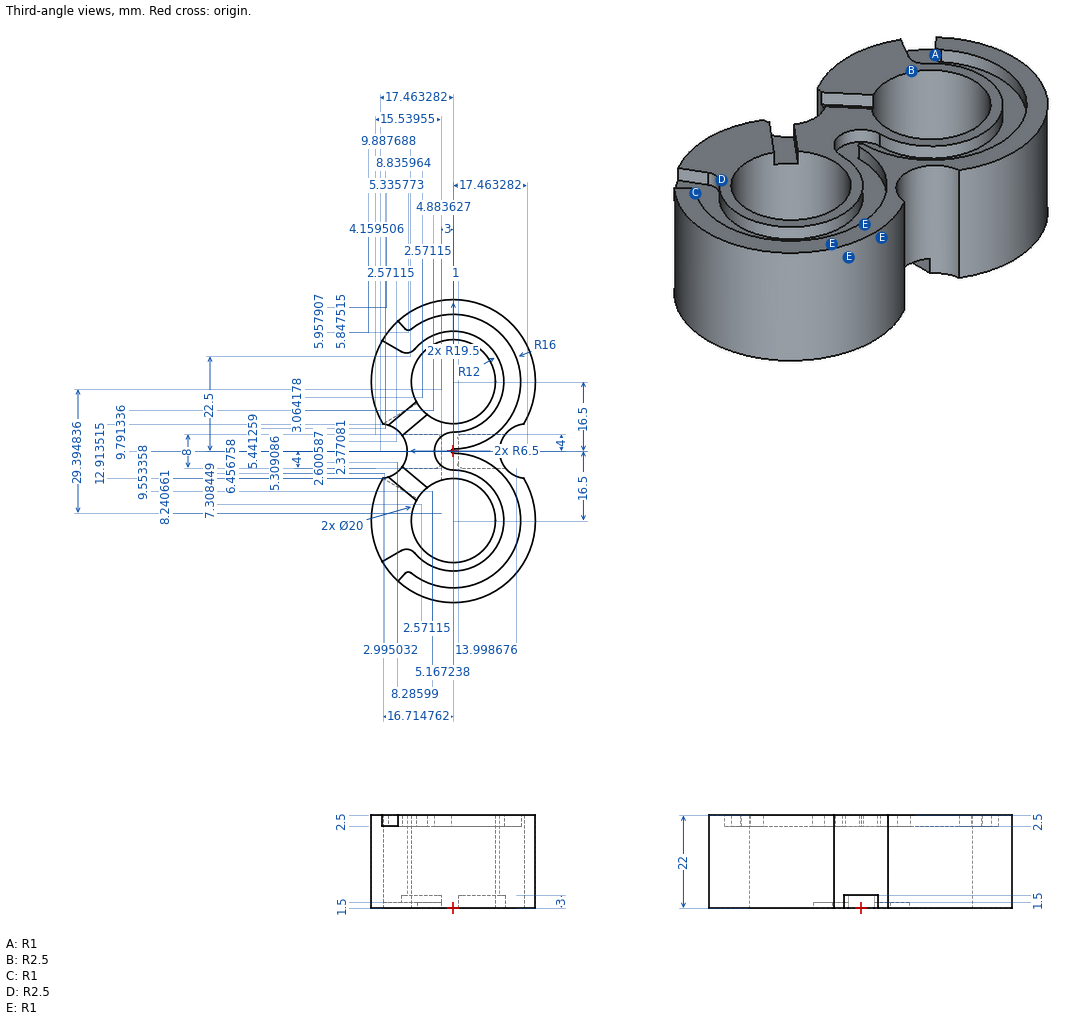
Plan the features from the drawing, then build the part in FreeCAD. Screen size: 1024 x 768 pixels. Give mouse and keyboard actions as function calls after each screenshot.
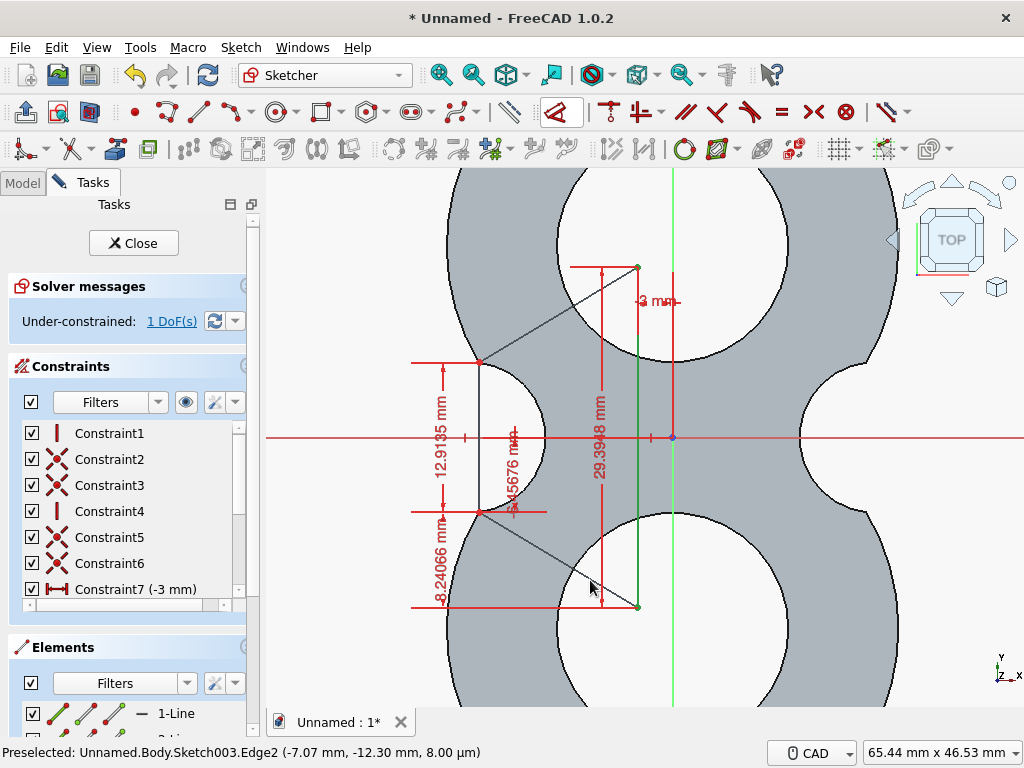
click(479, 512)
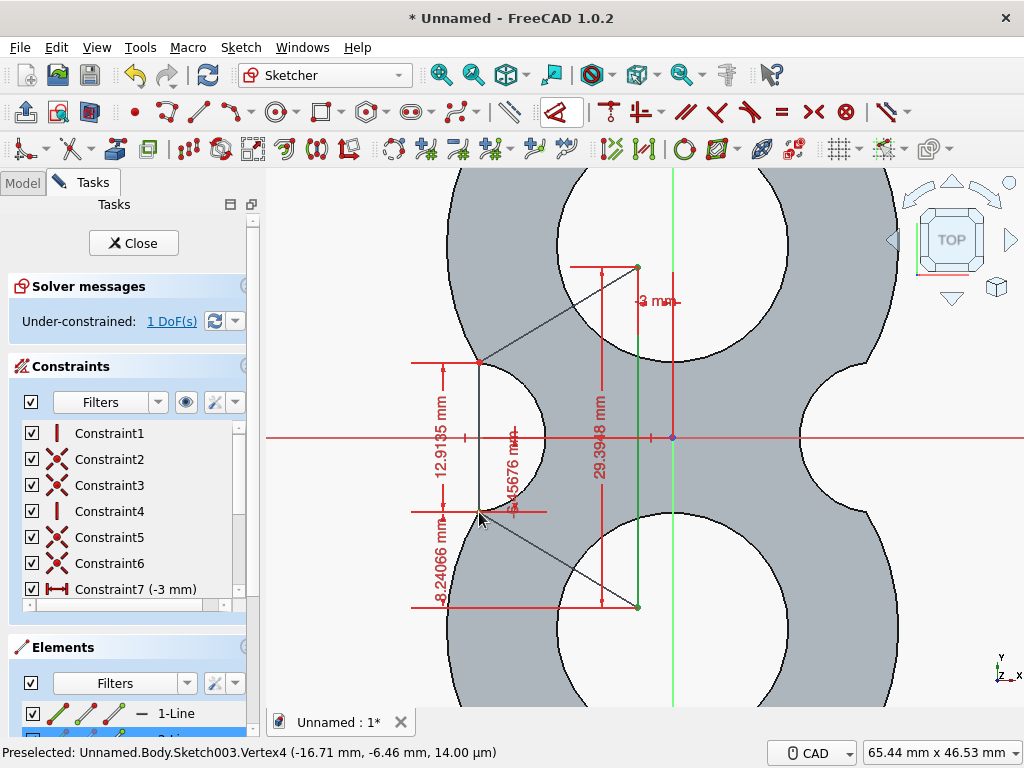
key(l)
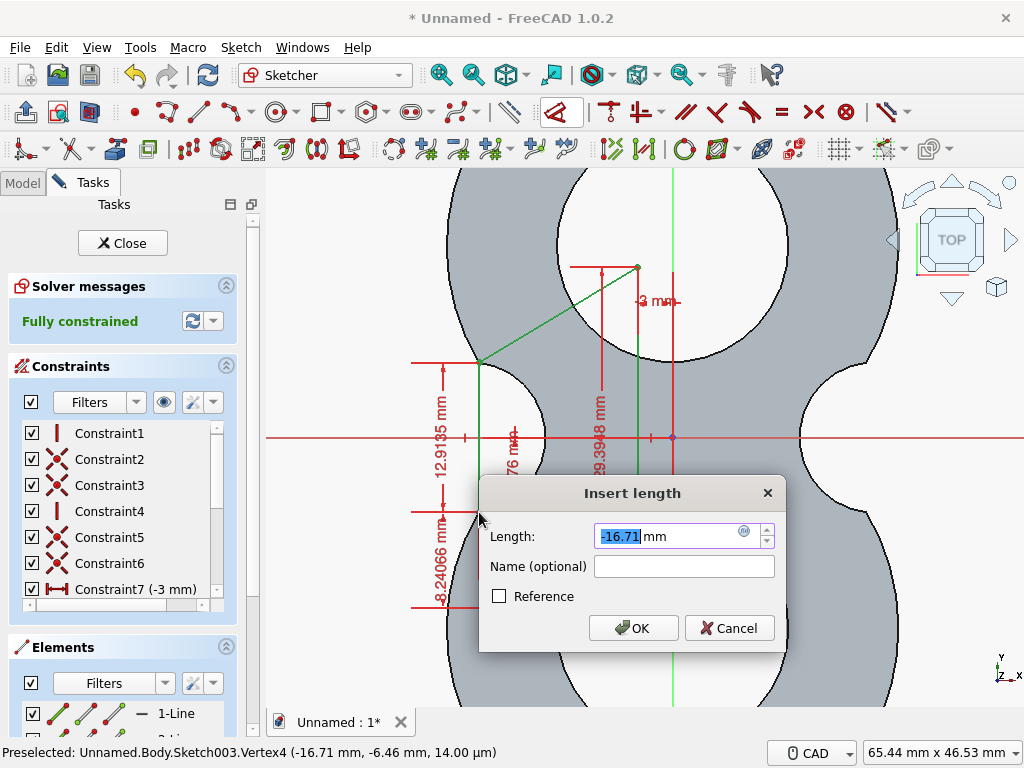
text(-16.714762)
key(Return)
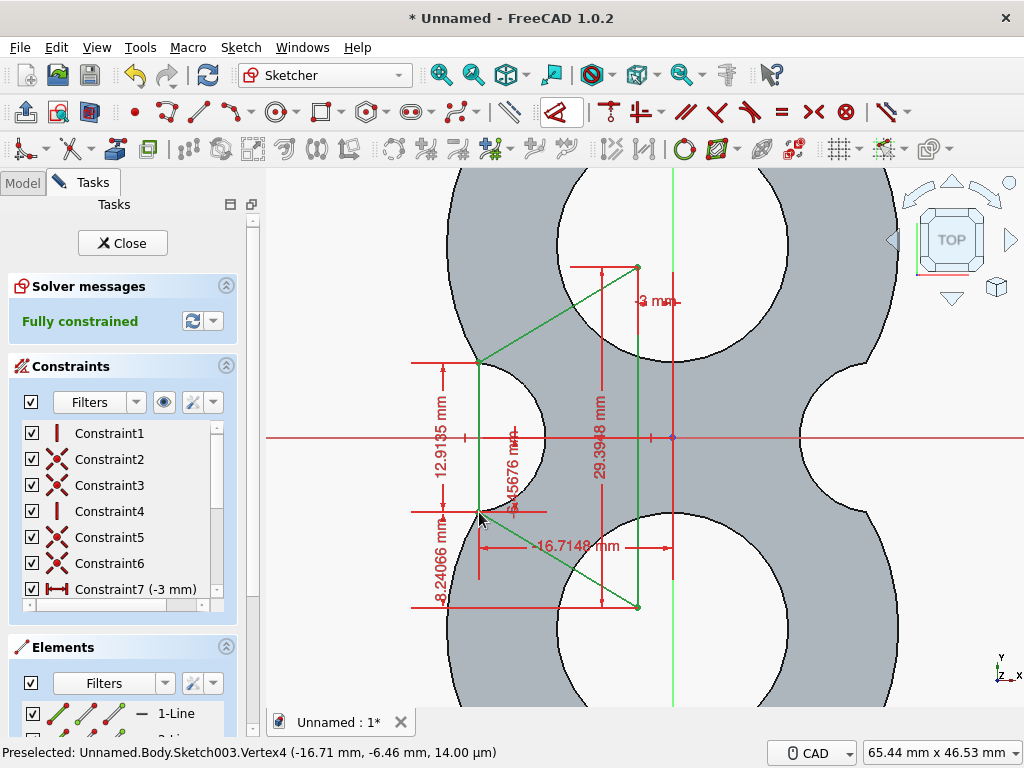
click(123, 243)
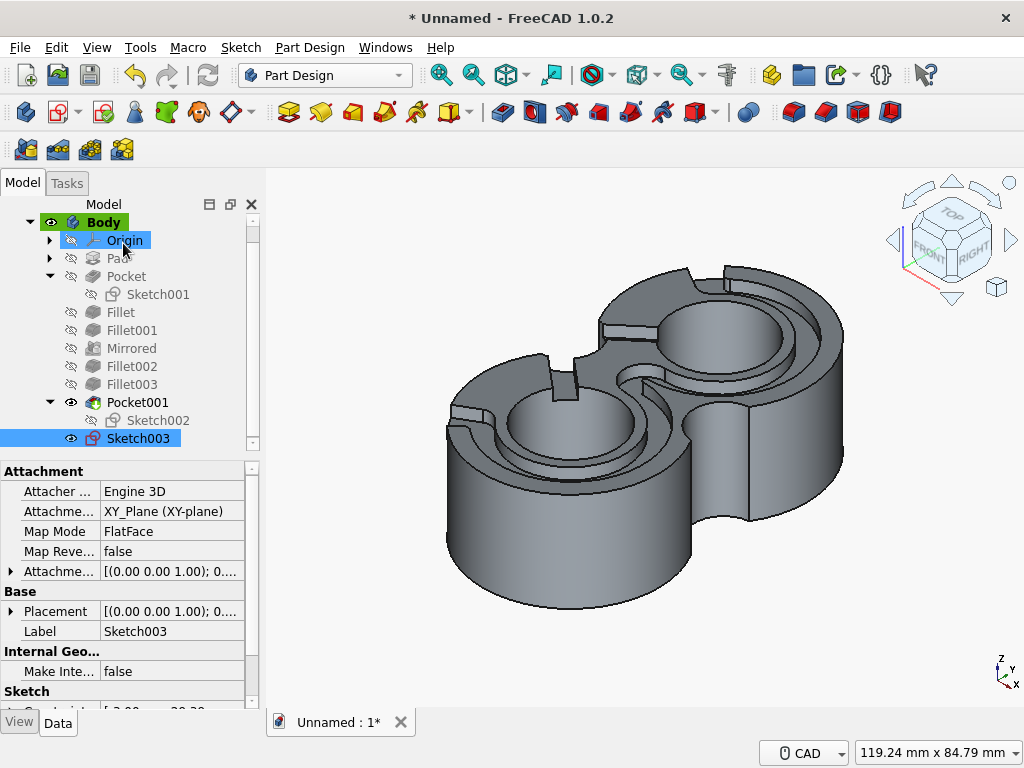
click(504, 112)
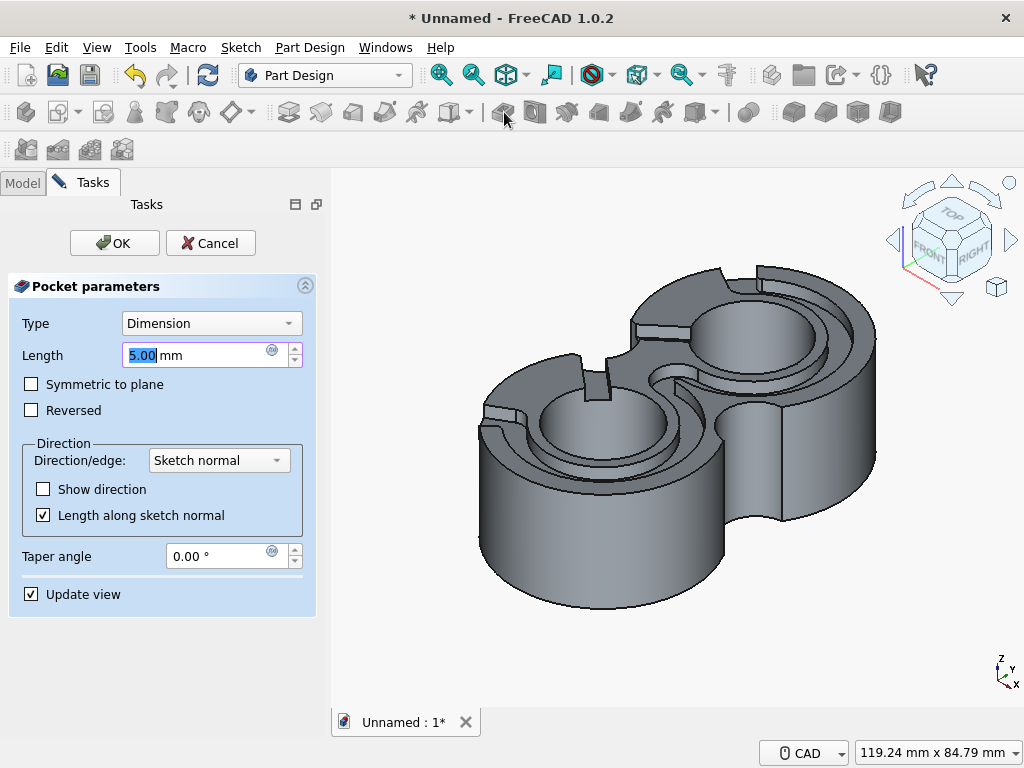
text(1.5)
key(Tab)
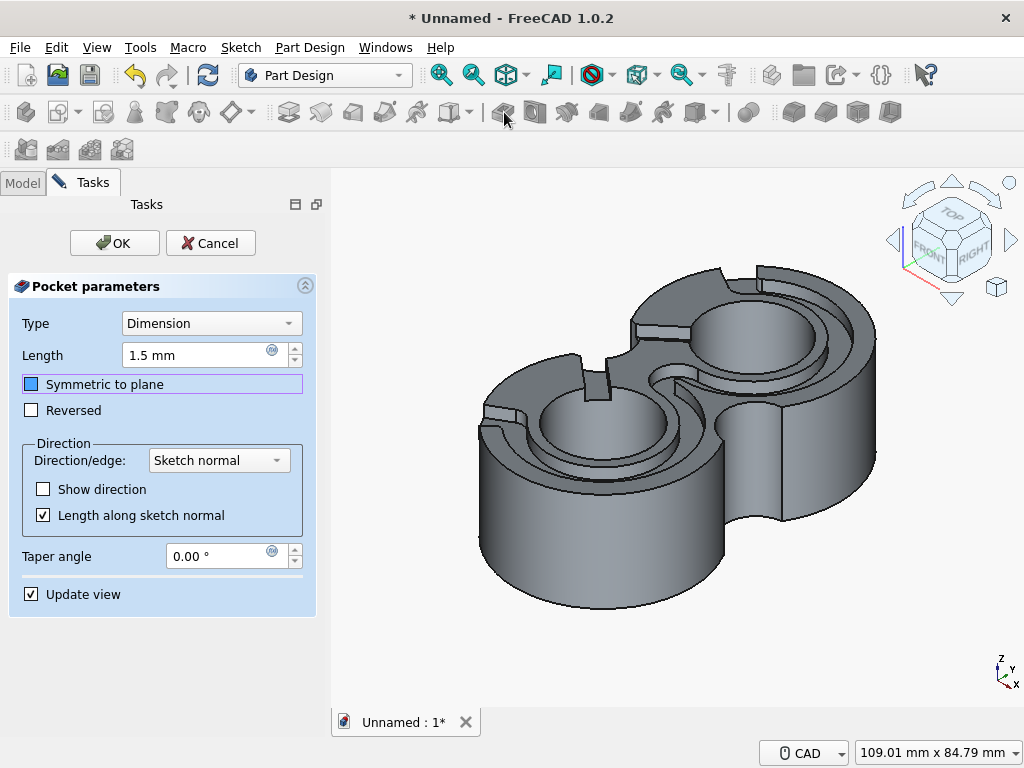
click(30, 410)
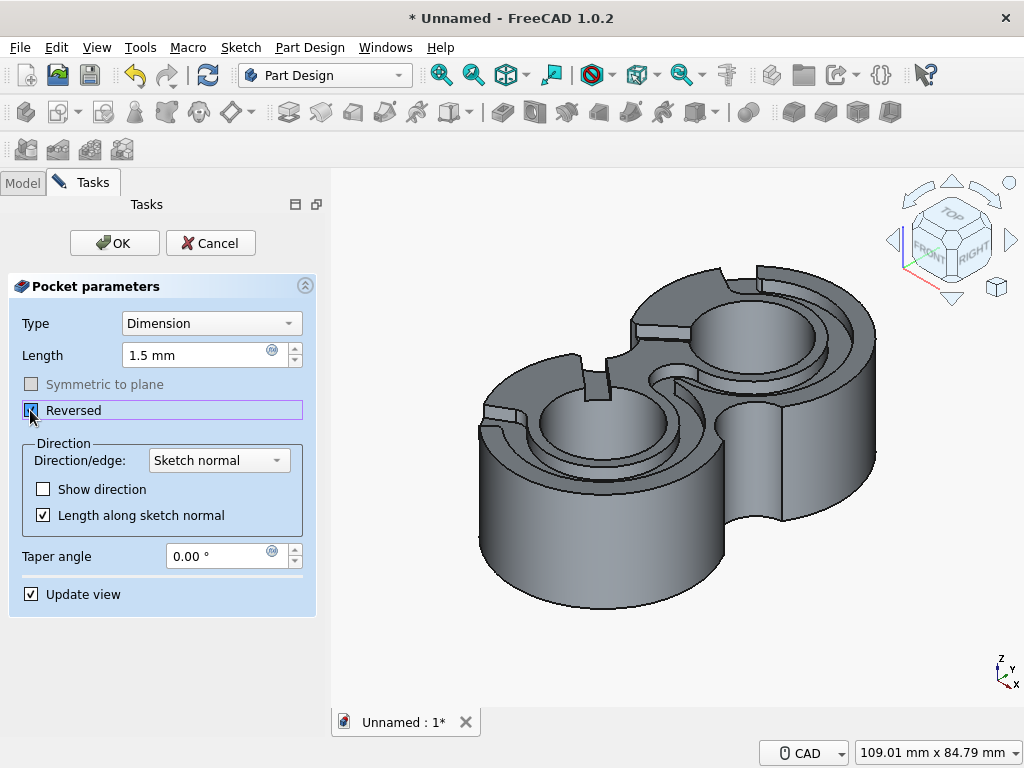
click(115, 243)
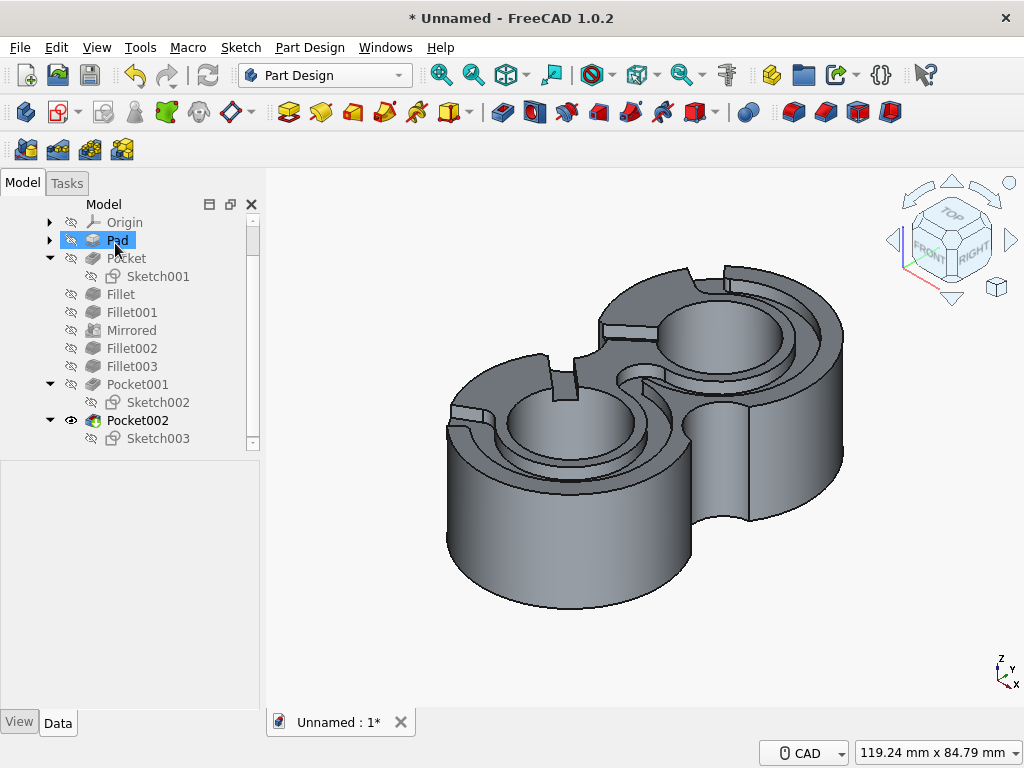
key(5)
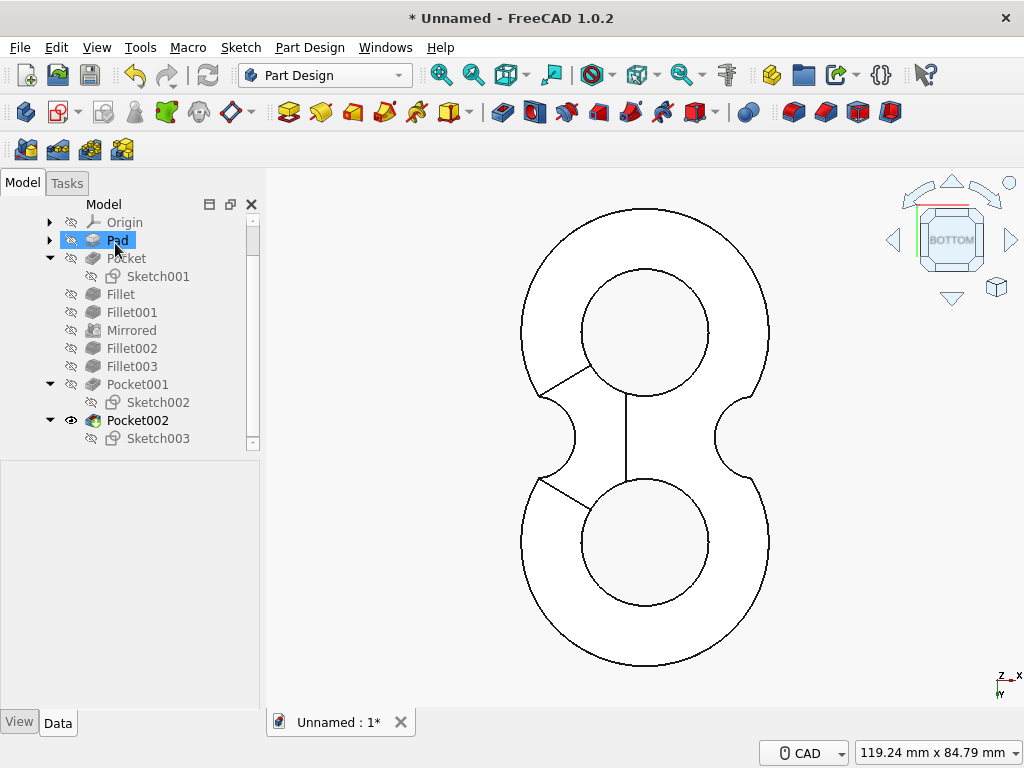
click(595, 416)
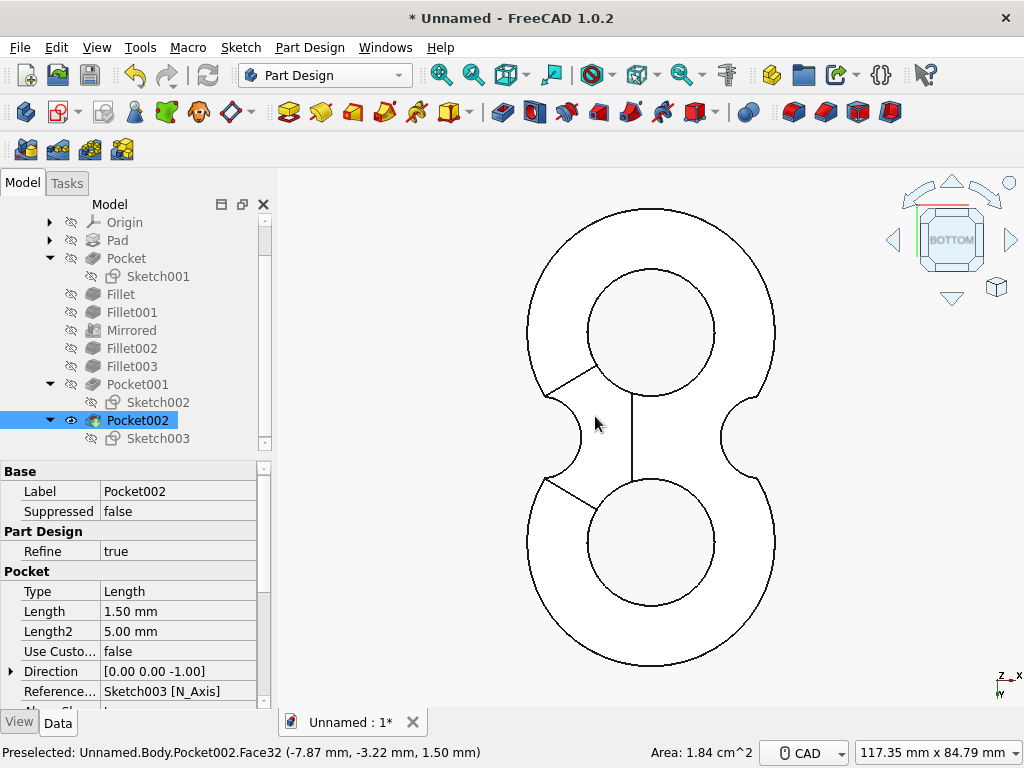
click(58, 112)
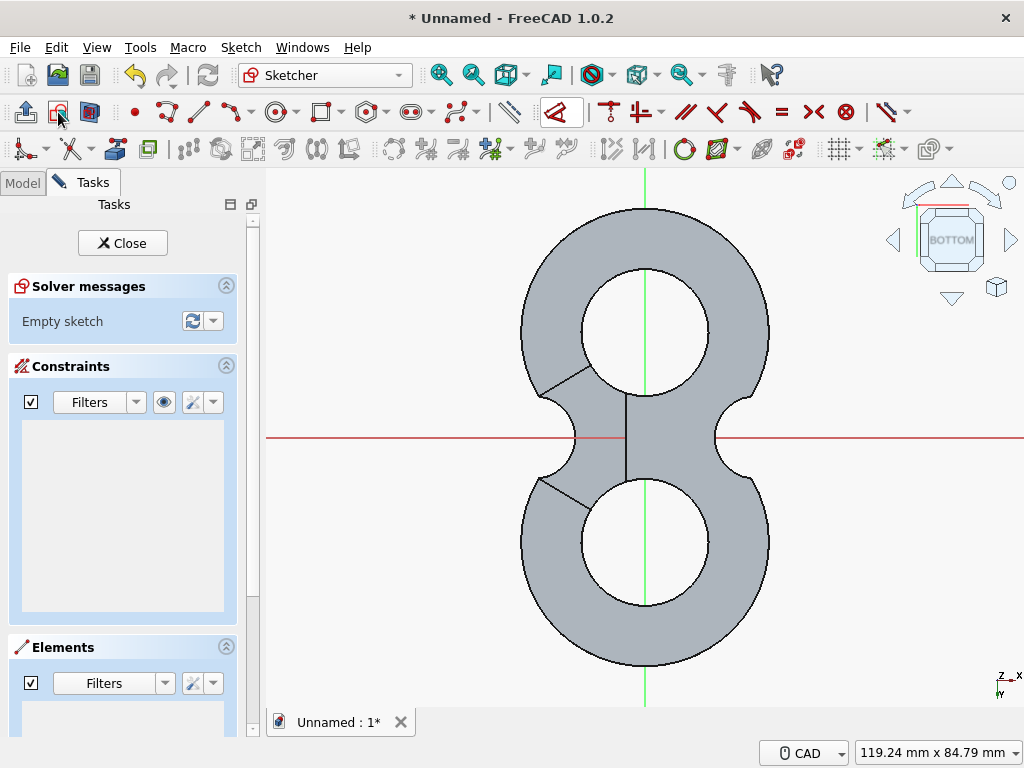
scroll(590, 438, up, 6)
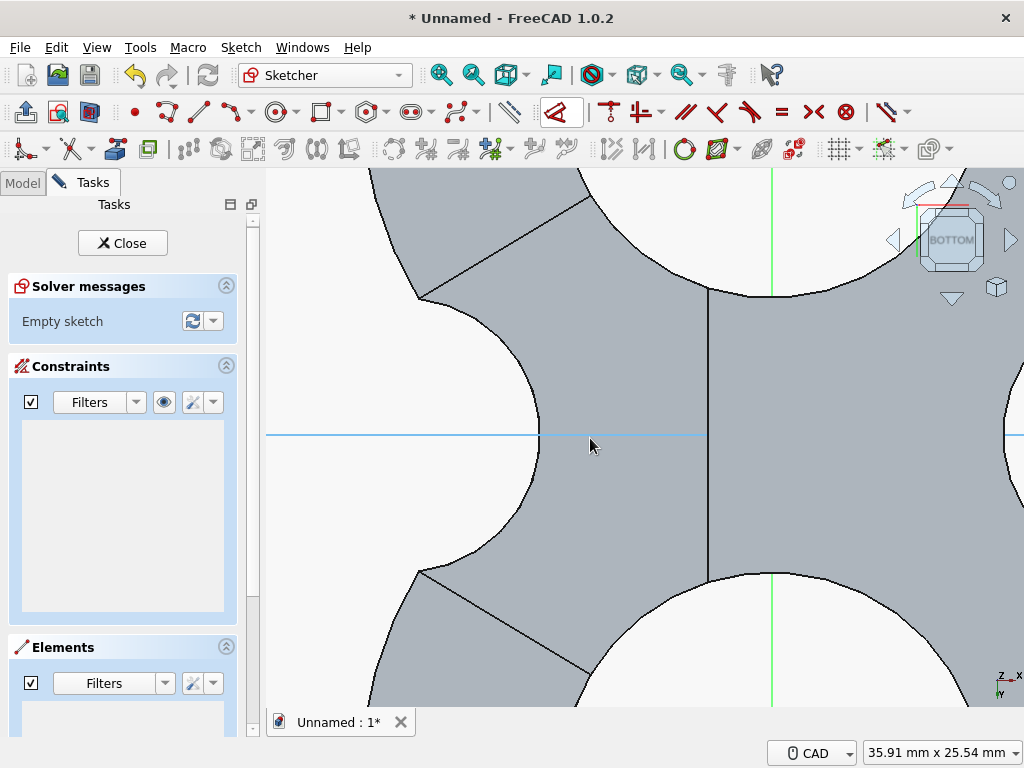
key(g)
key(r)